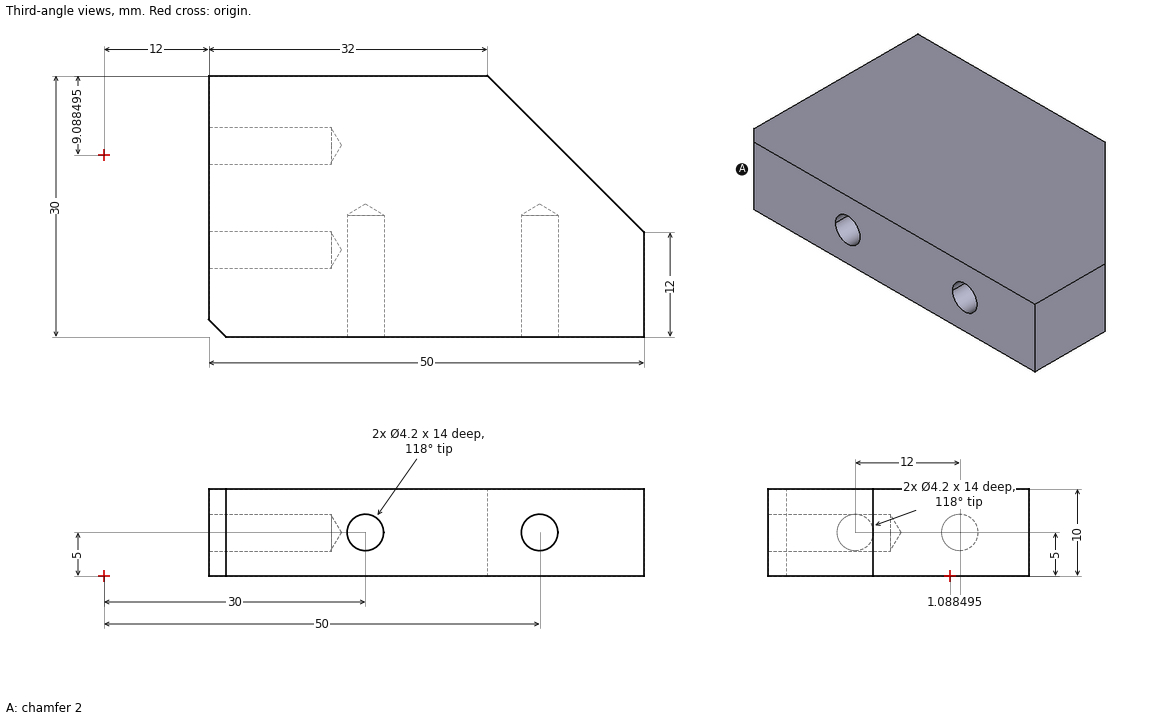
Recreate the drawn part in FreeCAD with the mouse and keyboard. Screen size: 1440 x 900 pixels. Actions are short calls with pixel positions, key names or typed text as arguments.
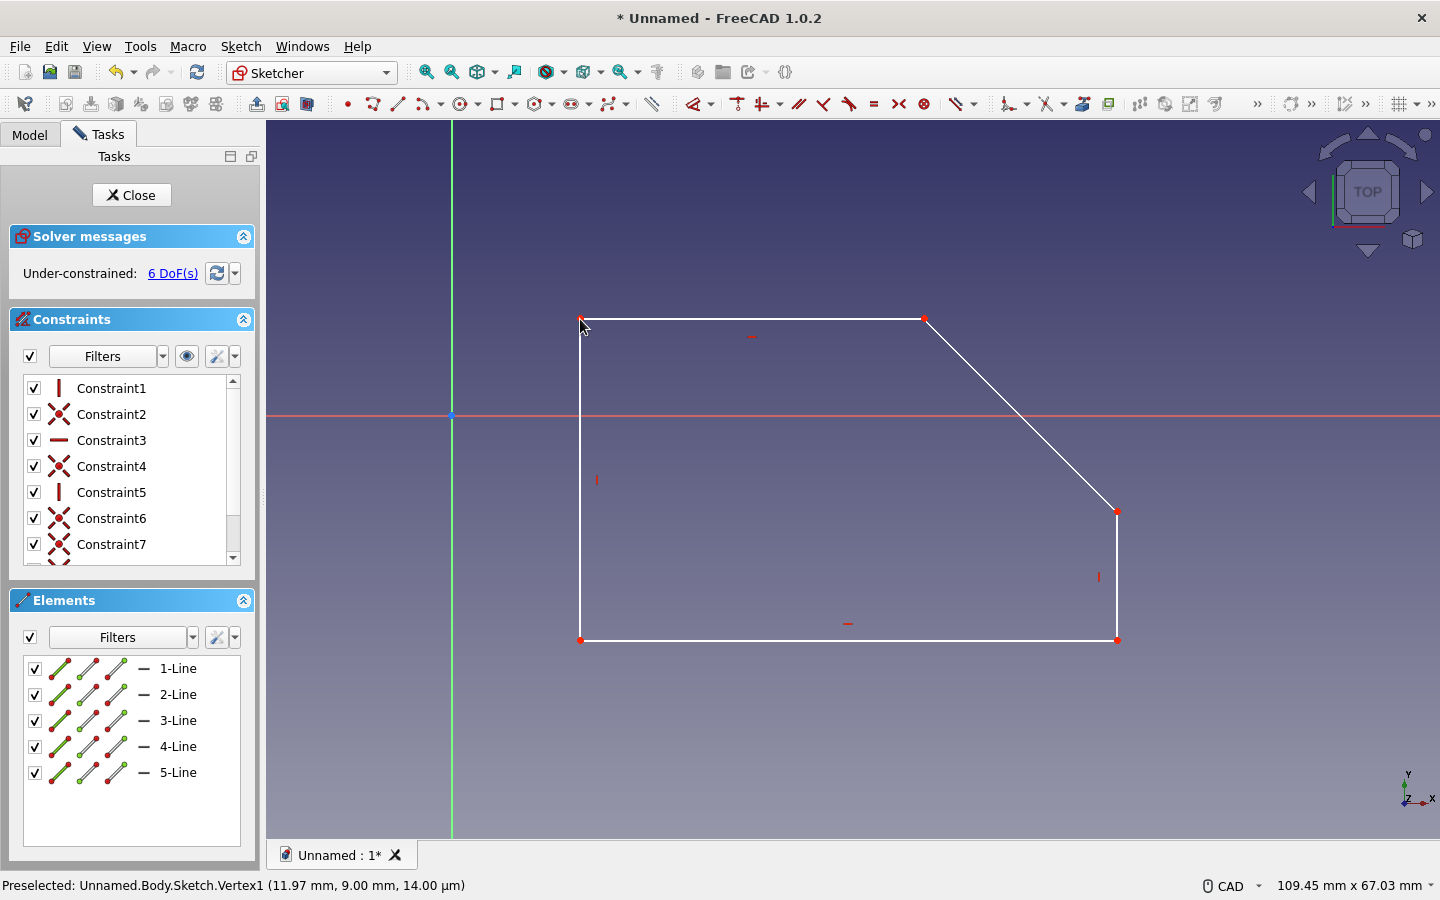
click(580, 416)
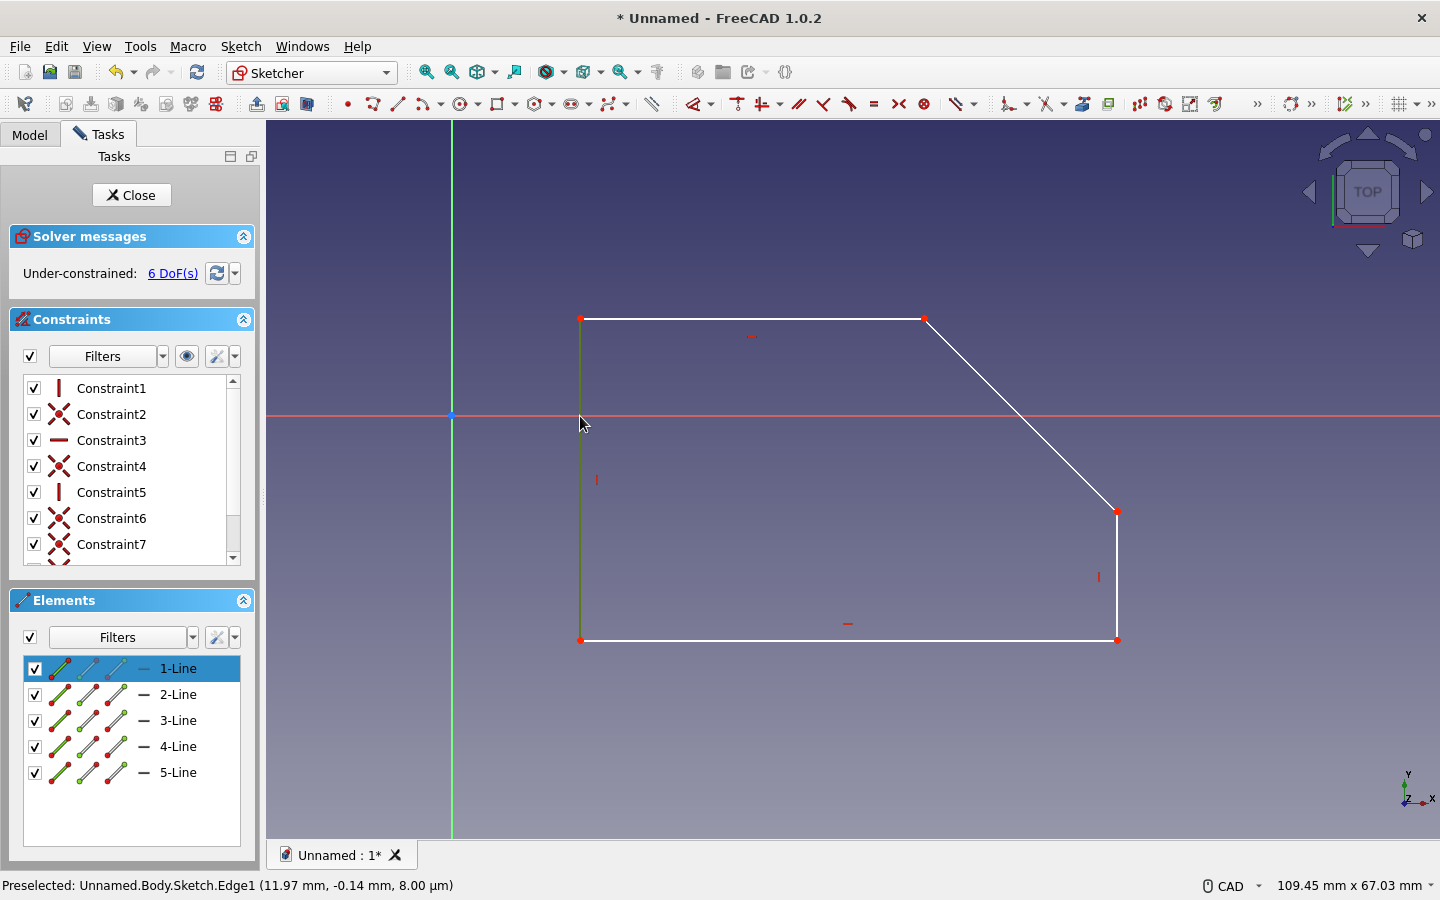
click(710, 104)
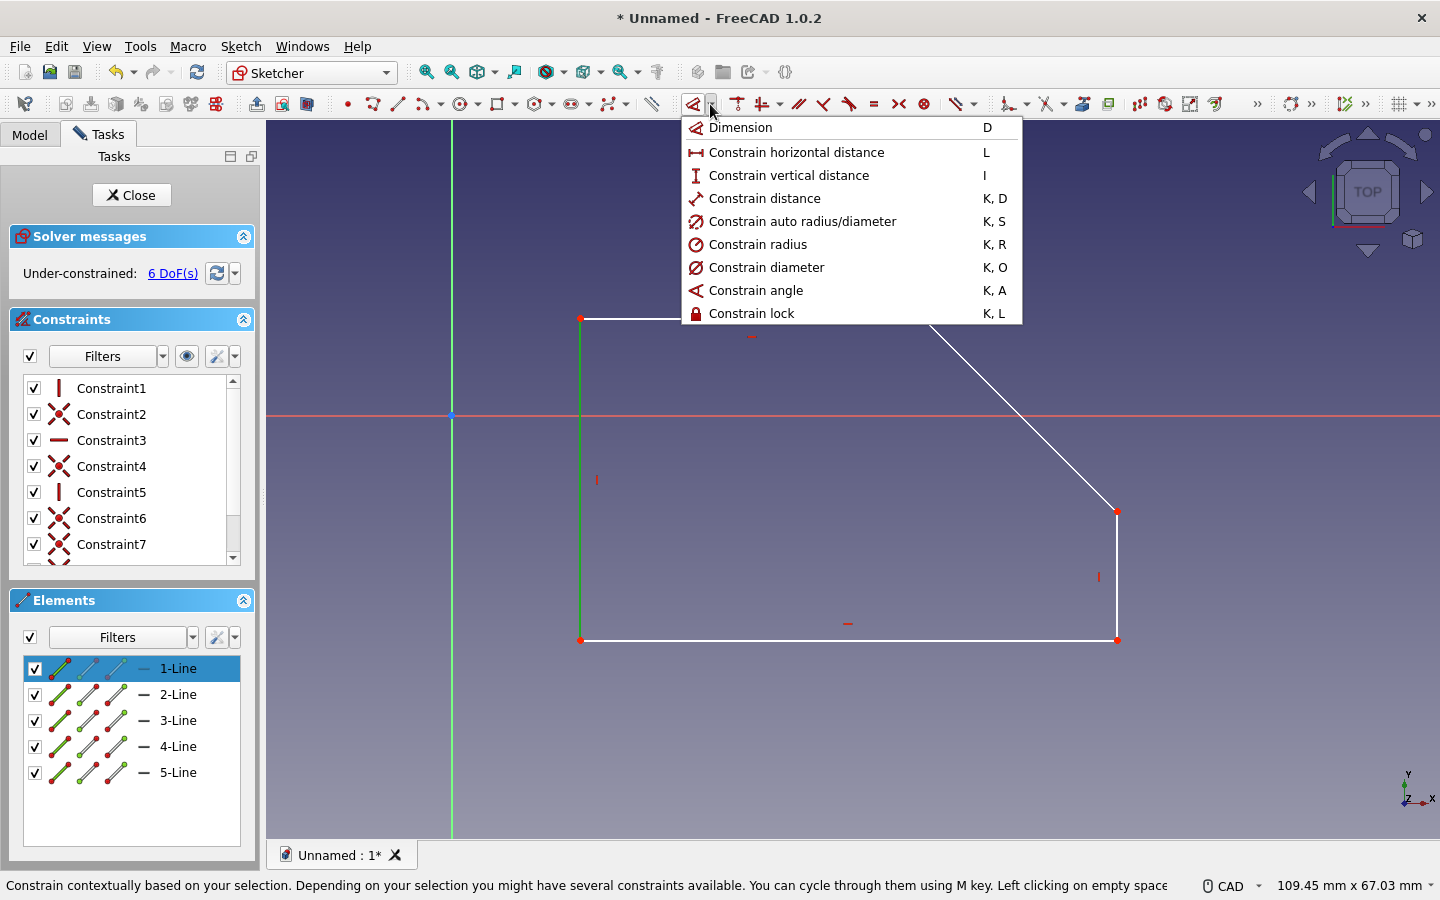
click(852, 176)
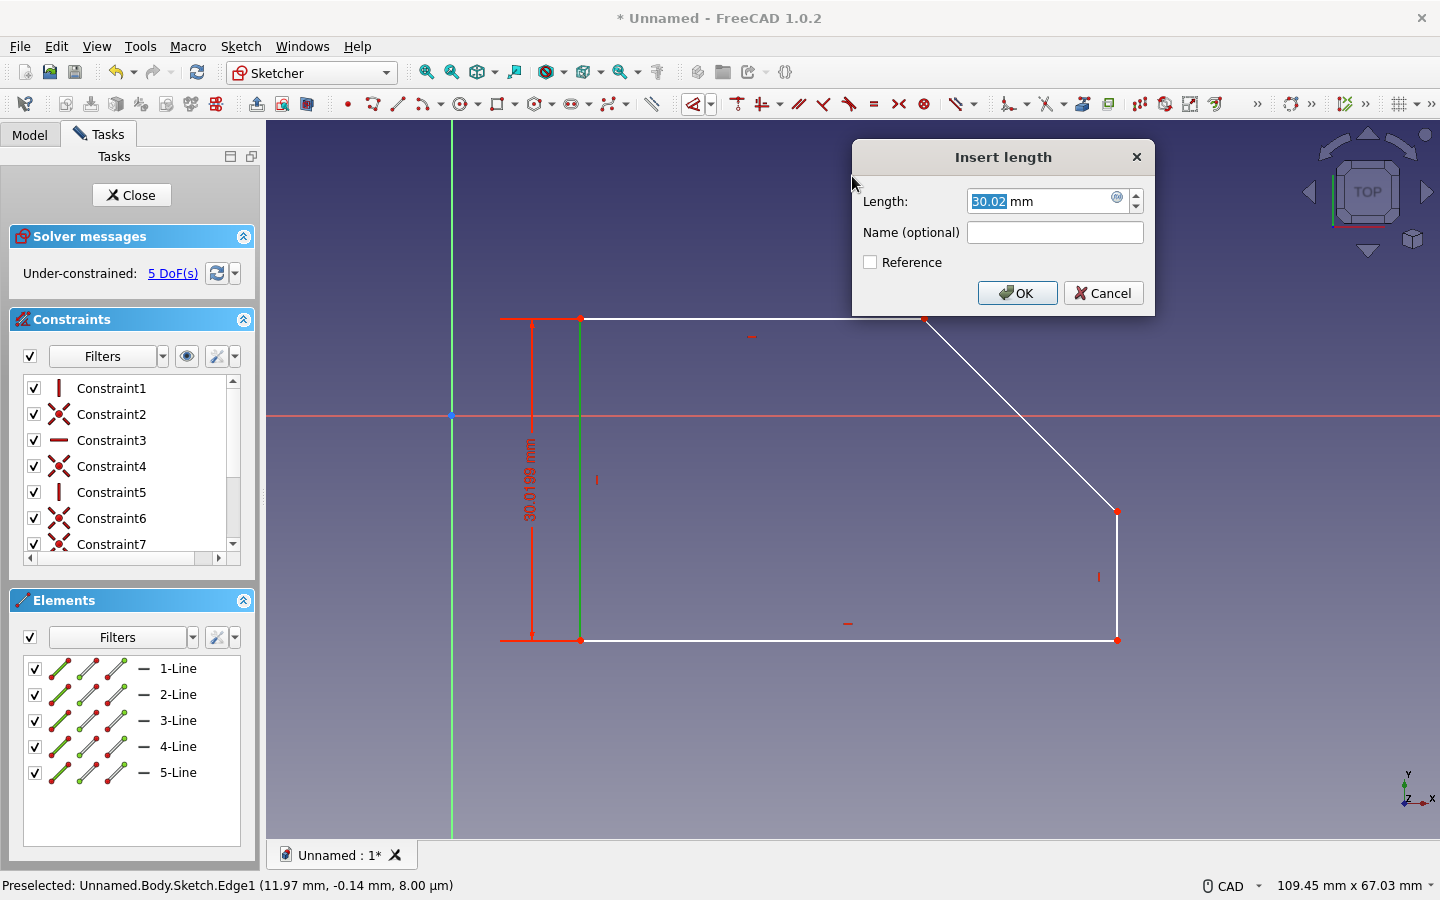
text(30)
key(Return)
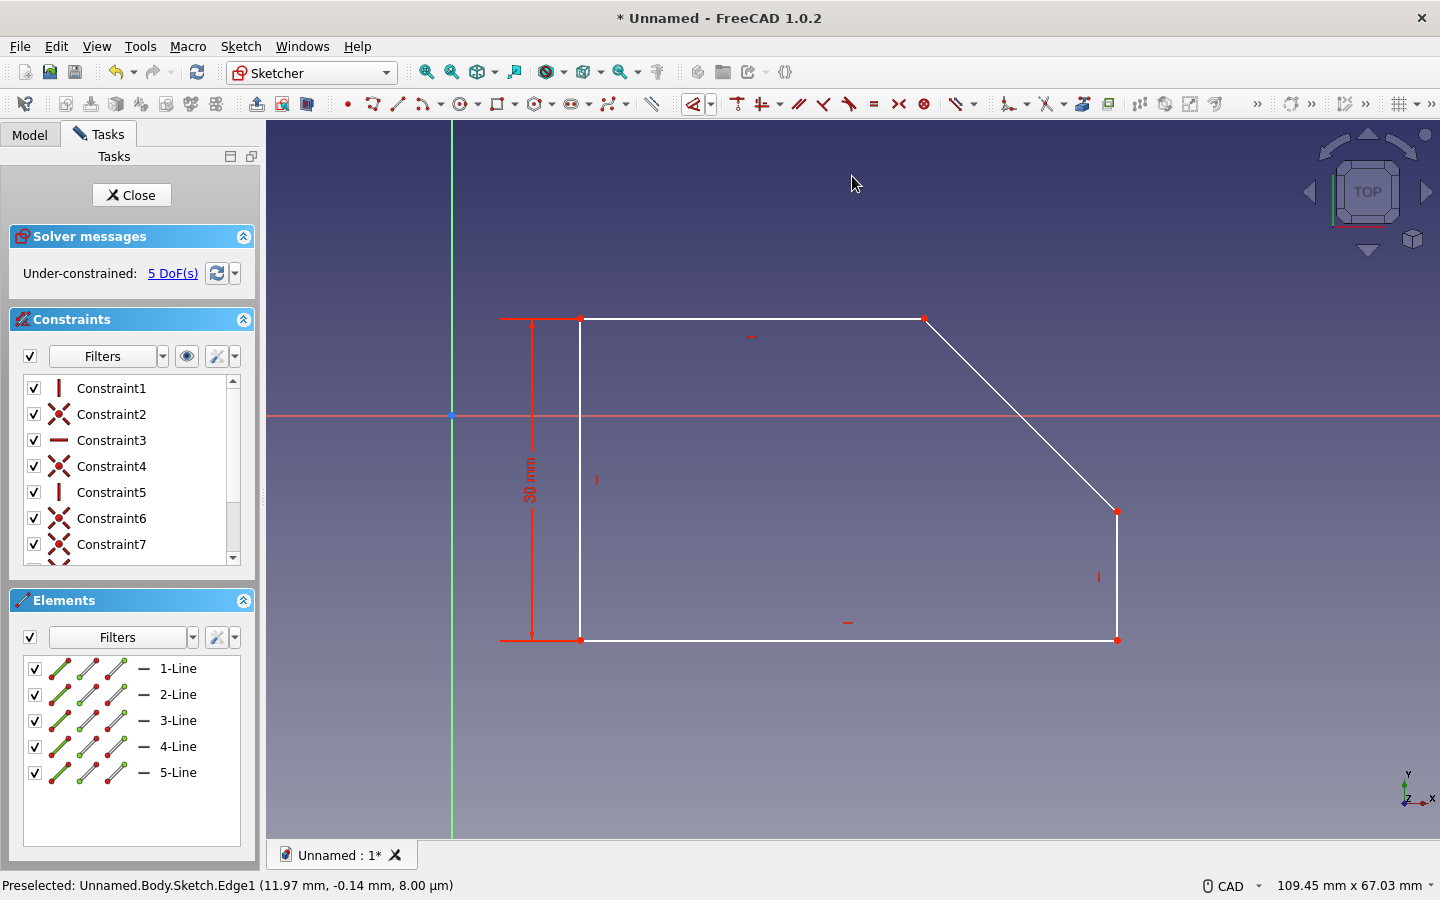
click(741, 641)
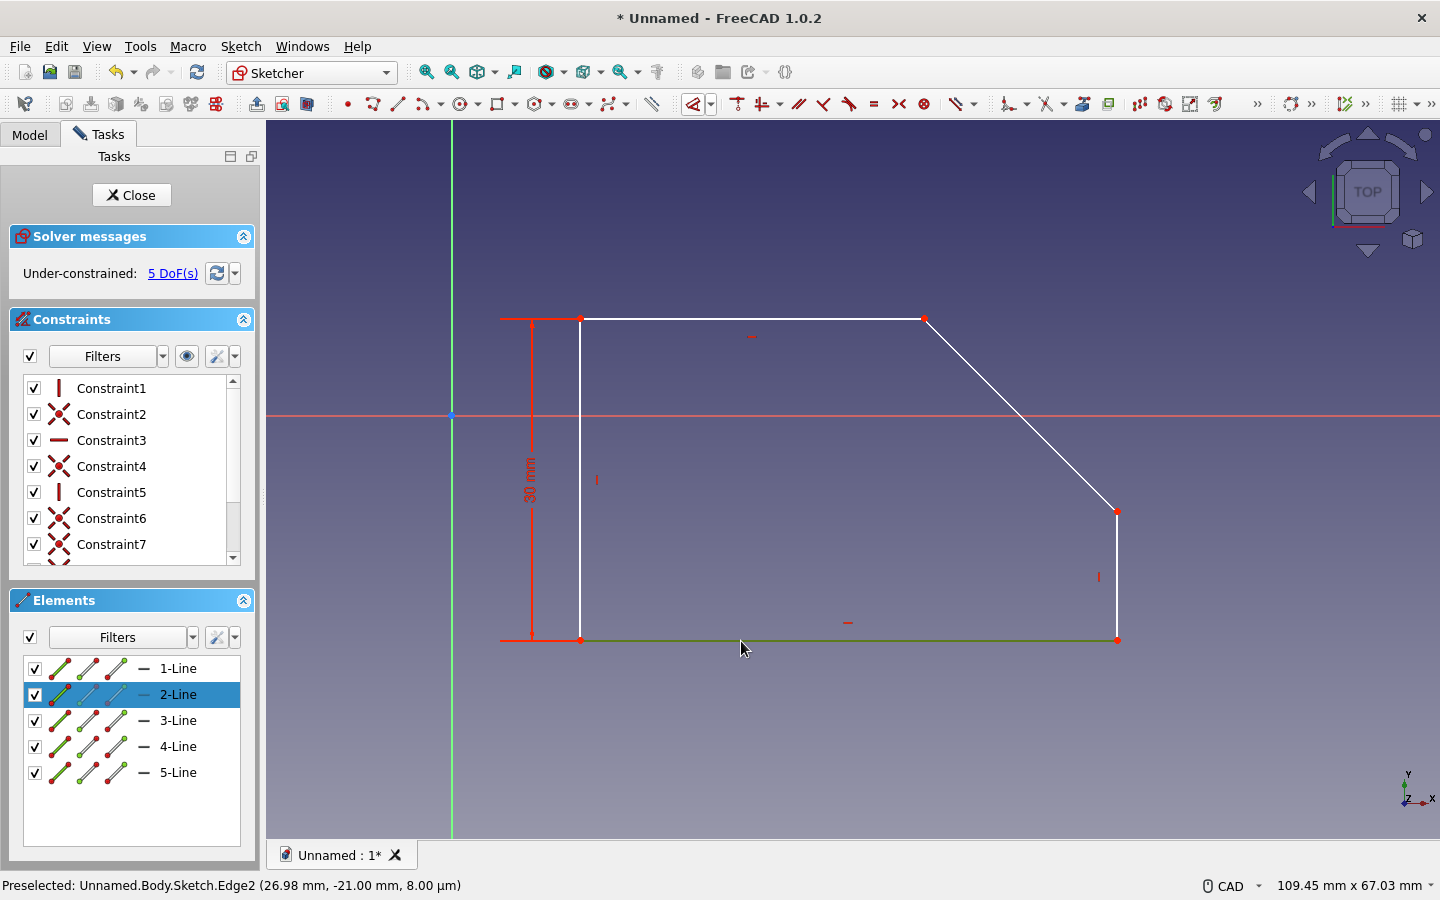
click(710, 104)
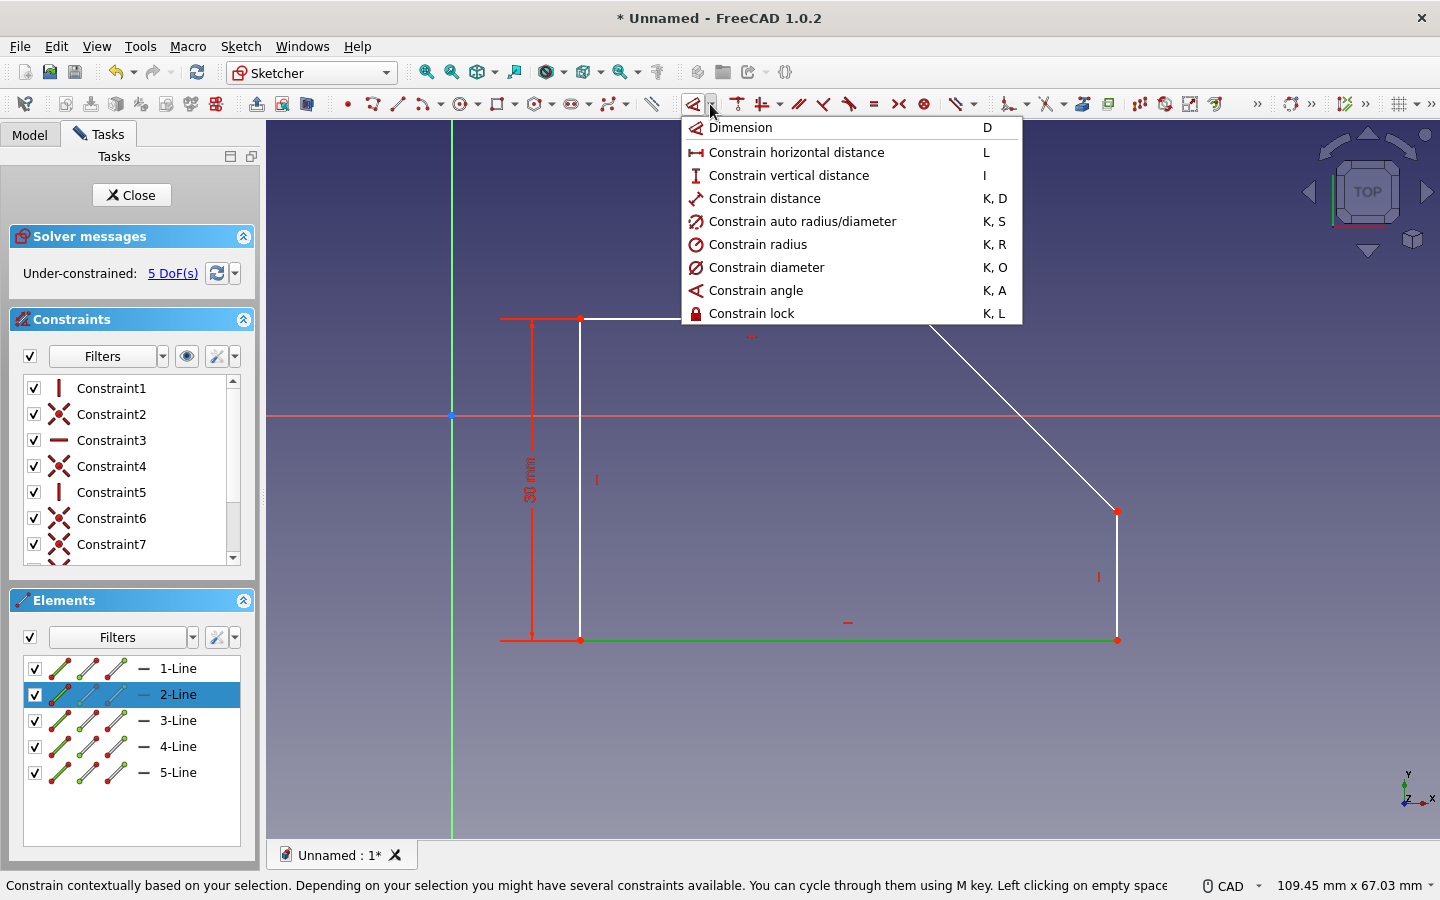
click(852, 152)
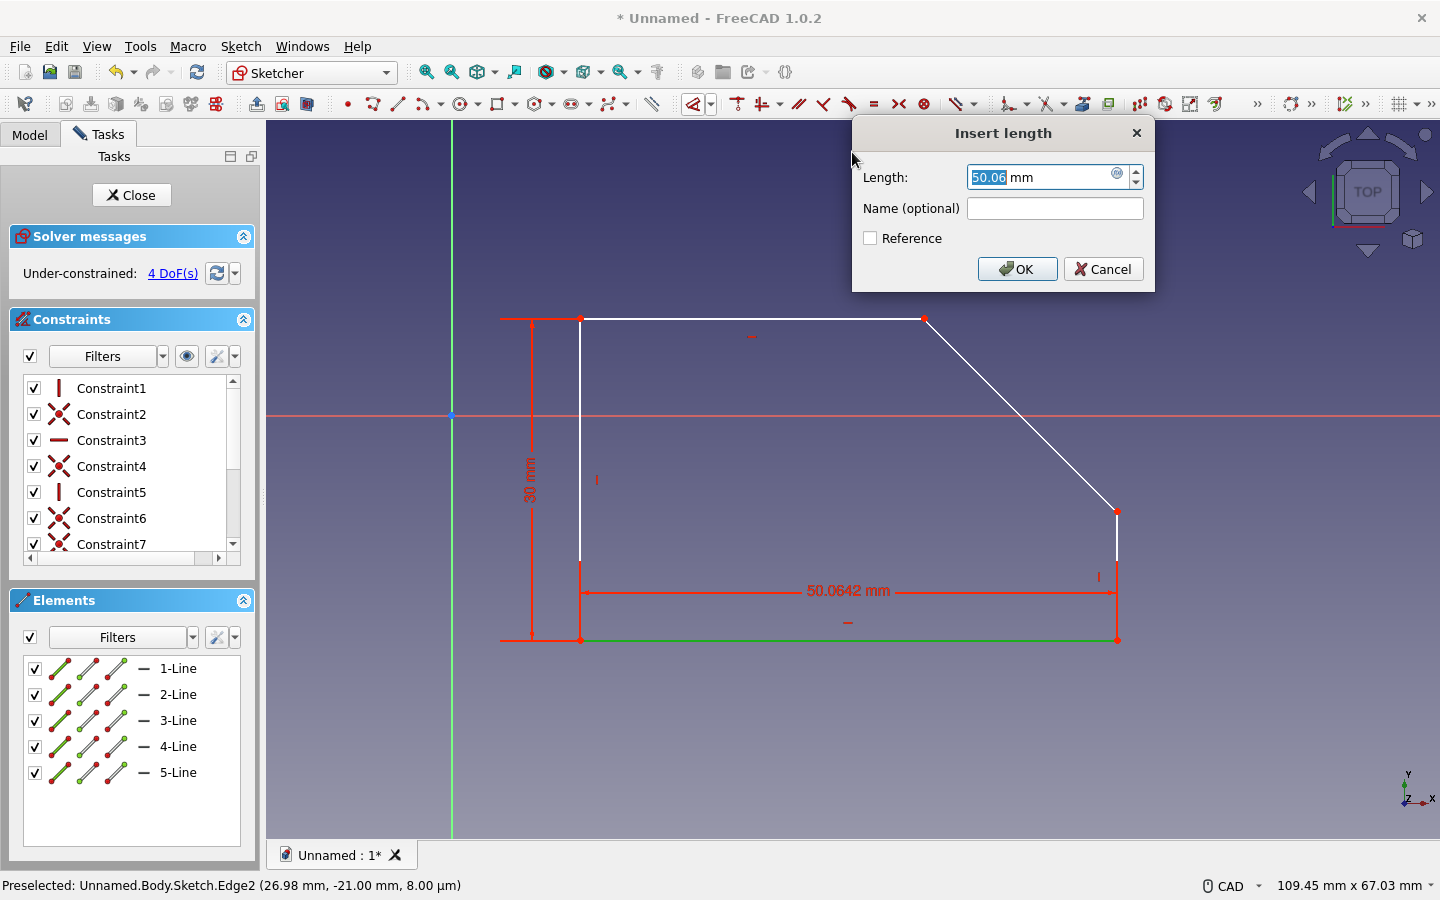
text(50)
key(Return)